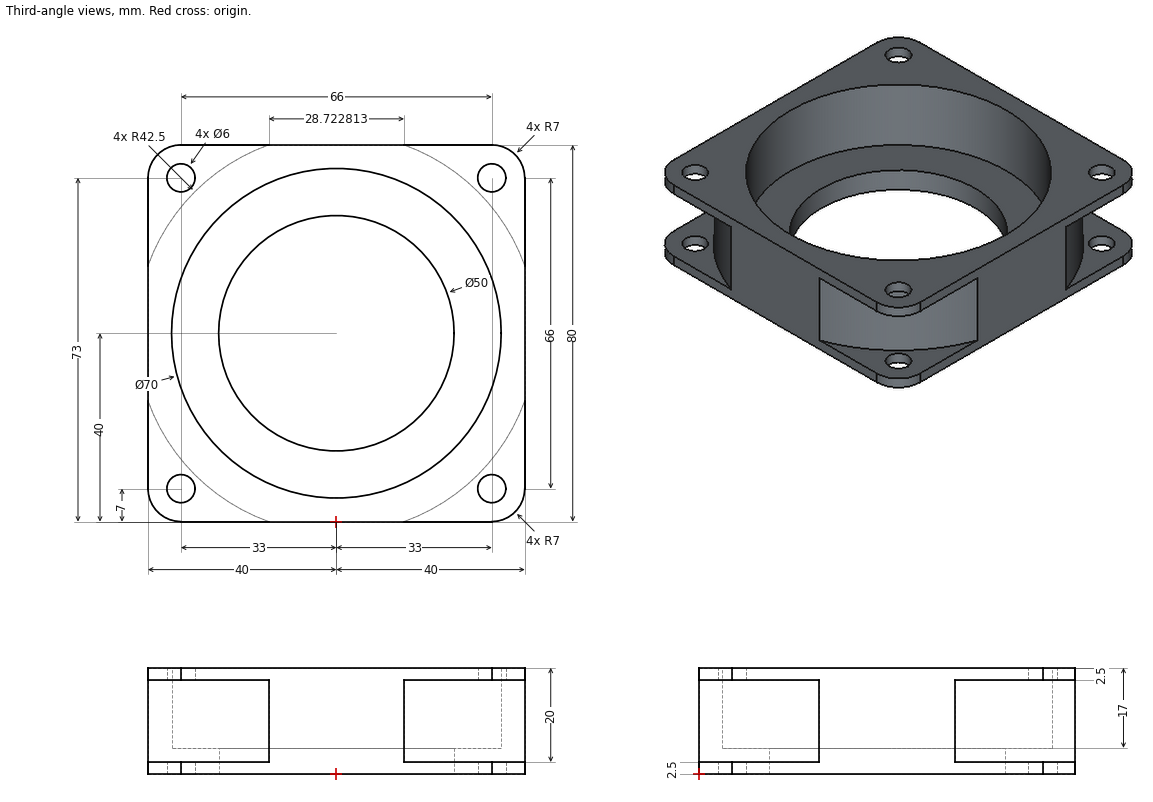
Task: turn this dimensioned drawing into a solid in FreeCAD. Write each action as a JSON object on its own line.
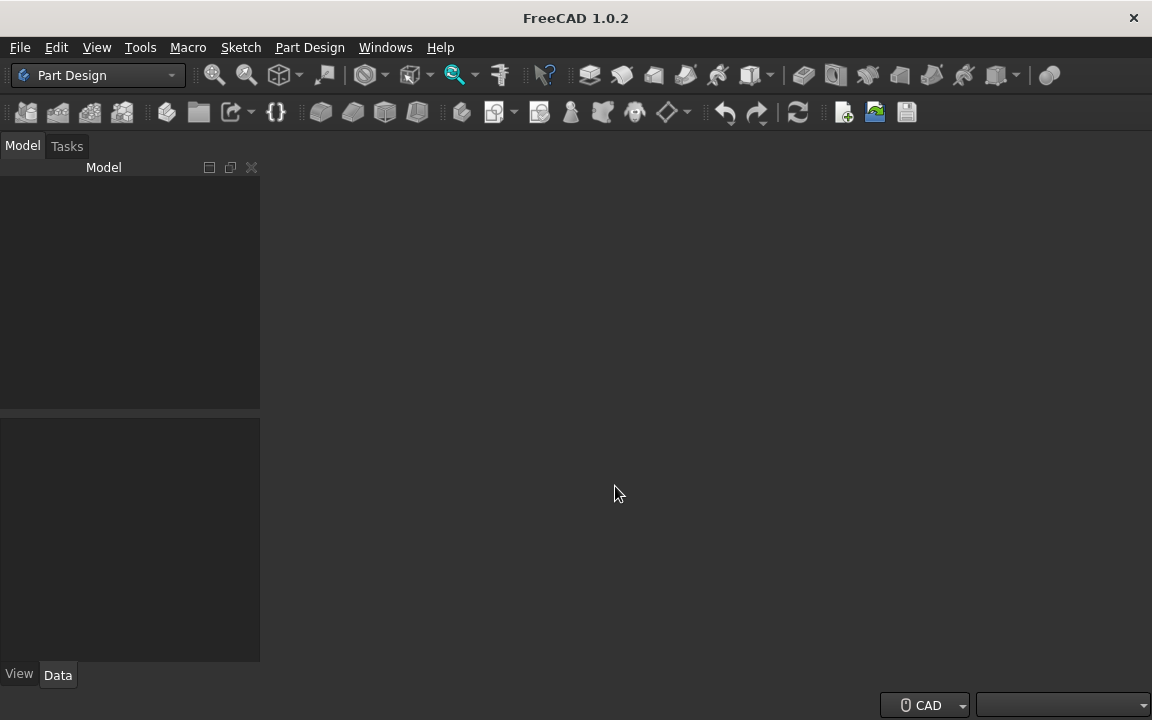
{"action": "left_click", "coordinate": [844, 112]}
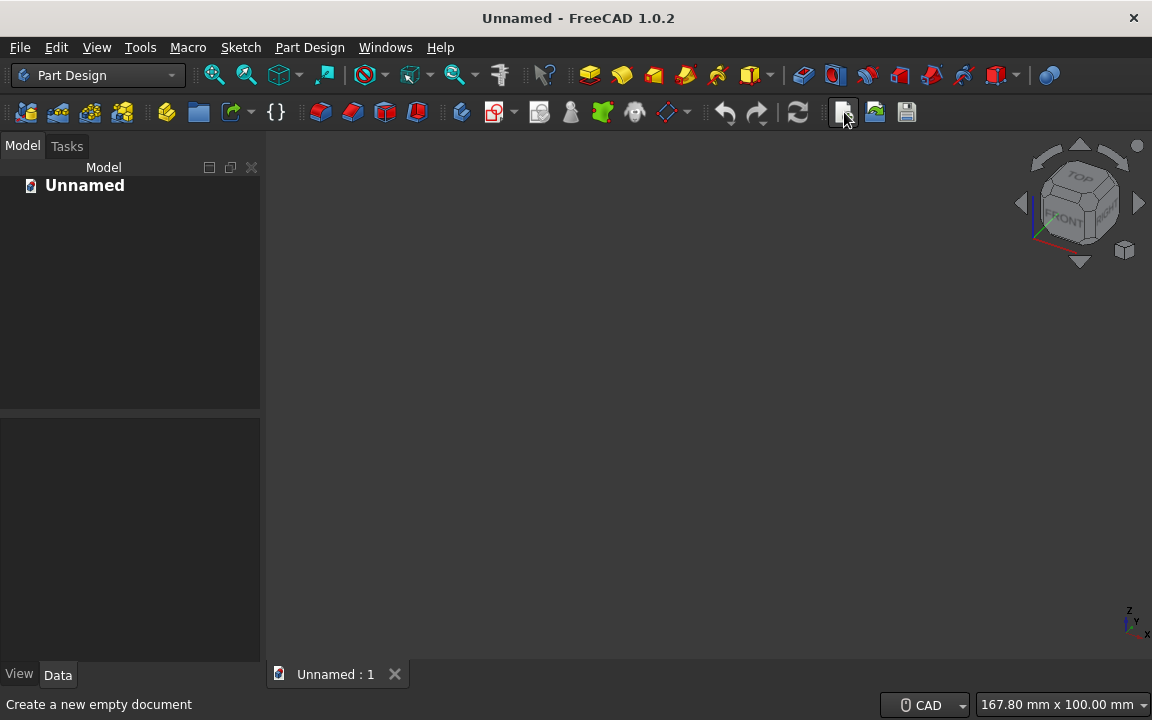
{"action": "left_click", "coordinate": [494, 112]}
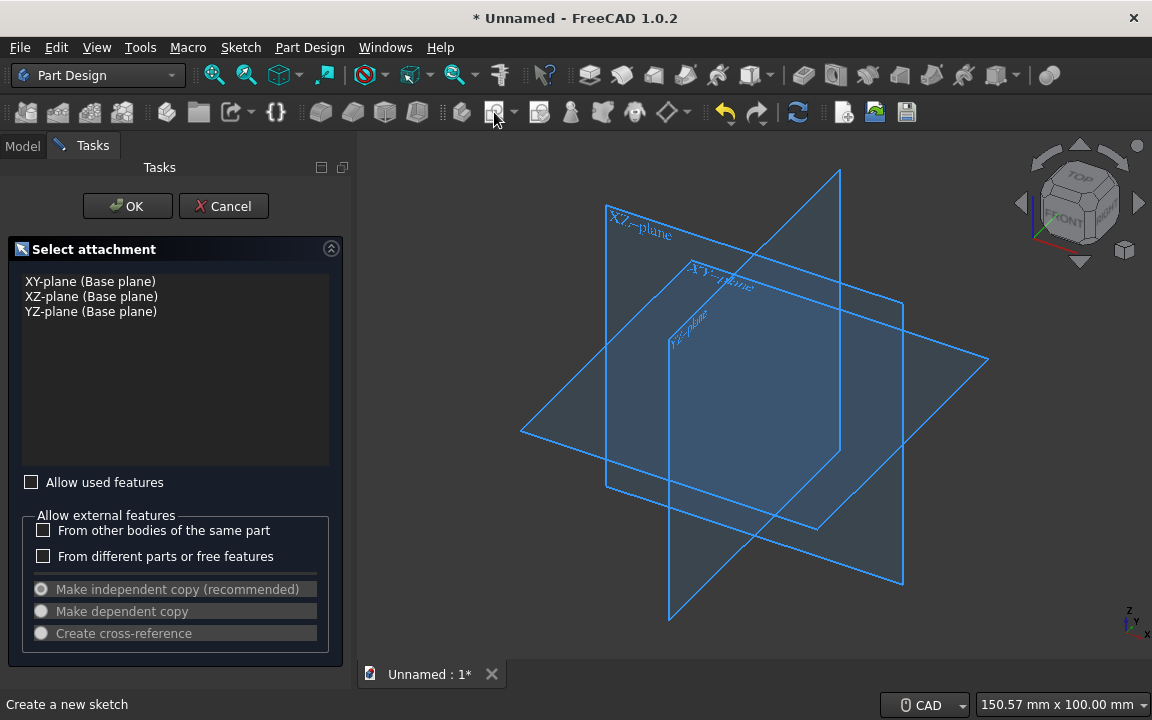
{"action": "left_click", "coordinate": [82, 282]}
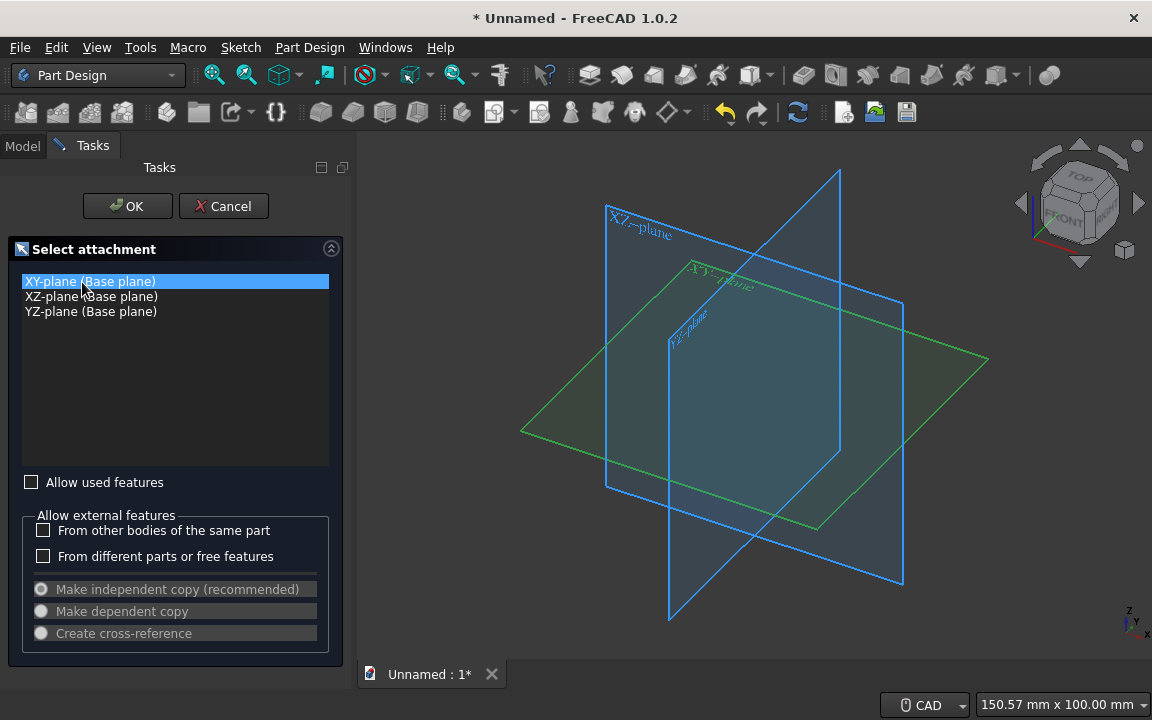
{"action": "left_click", "coordinate": [128, 206]}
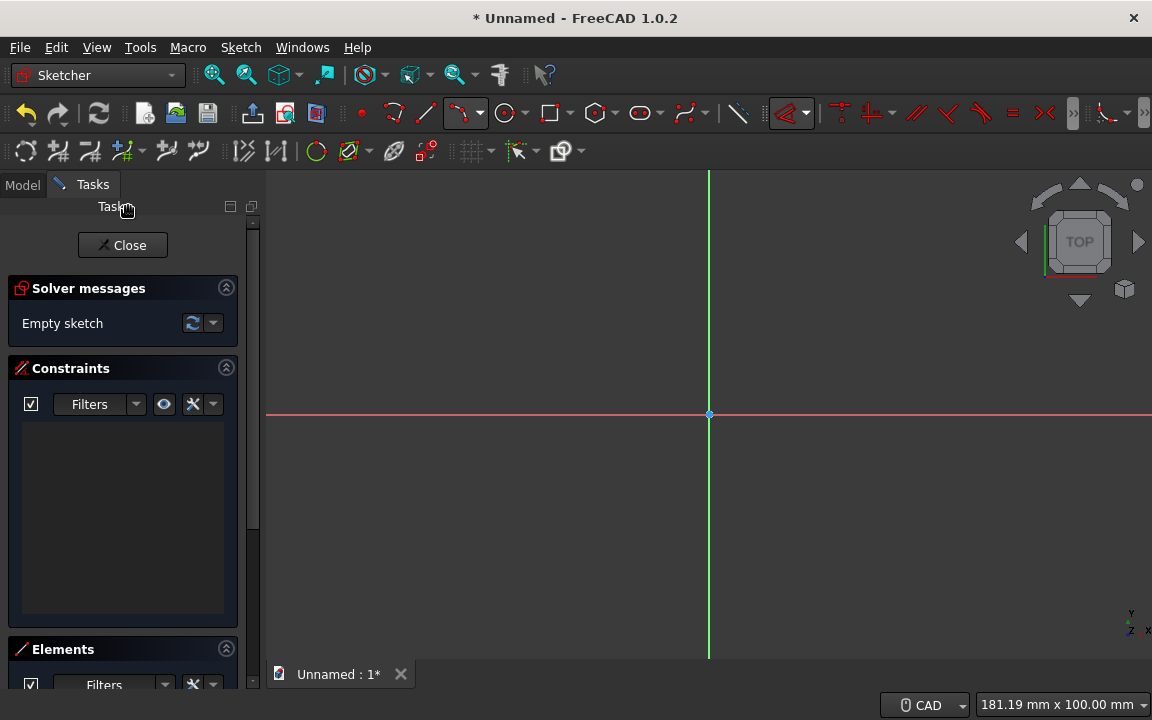
{"action": "scroll", "coordinate": [501, 631], "scroll_direction": "down", "scroll_amount": 2}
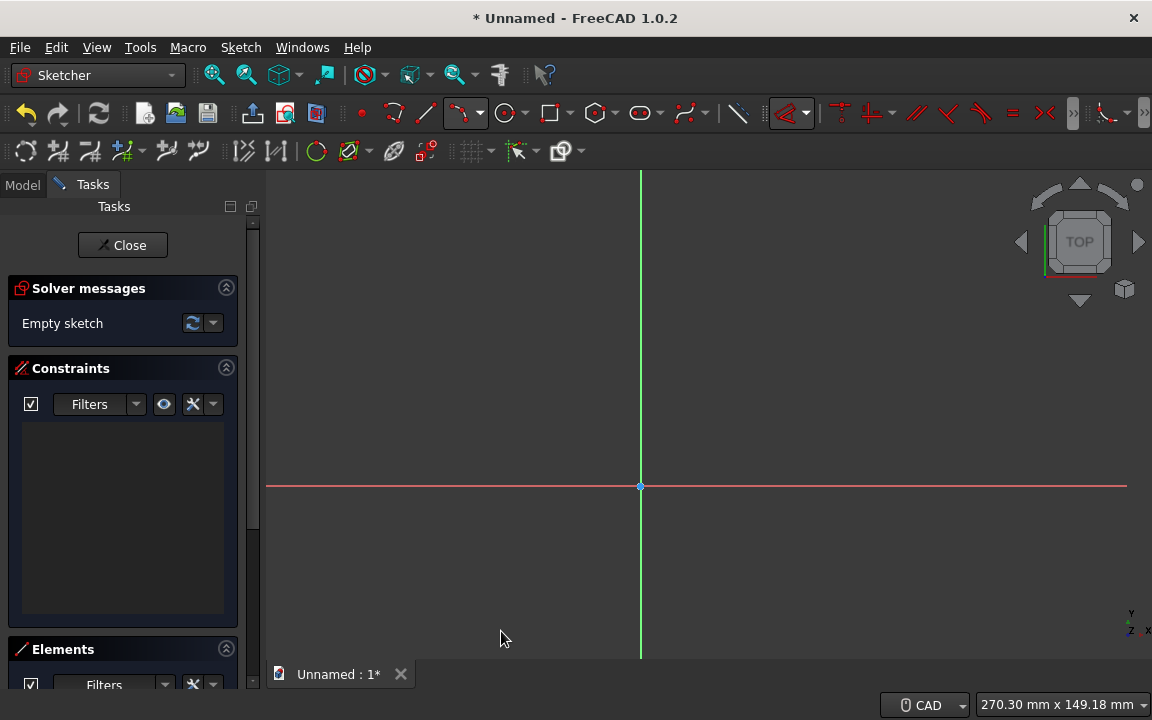
{"action": "left_click", "coordinate": [426, 114]}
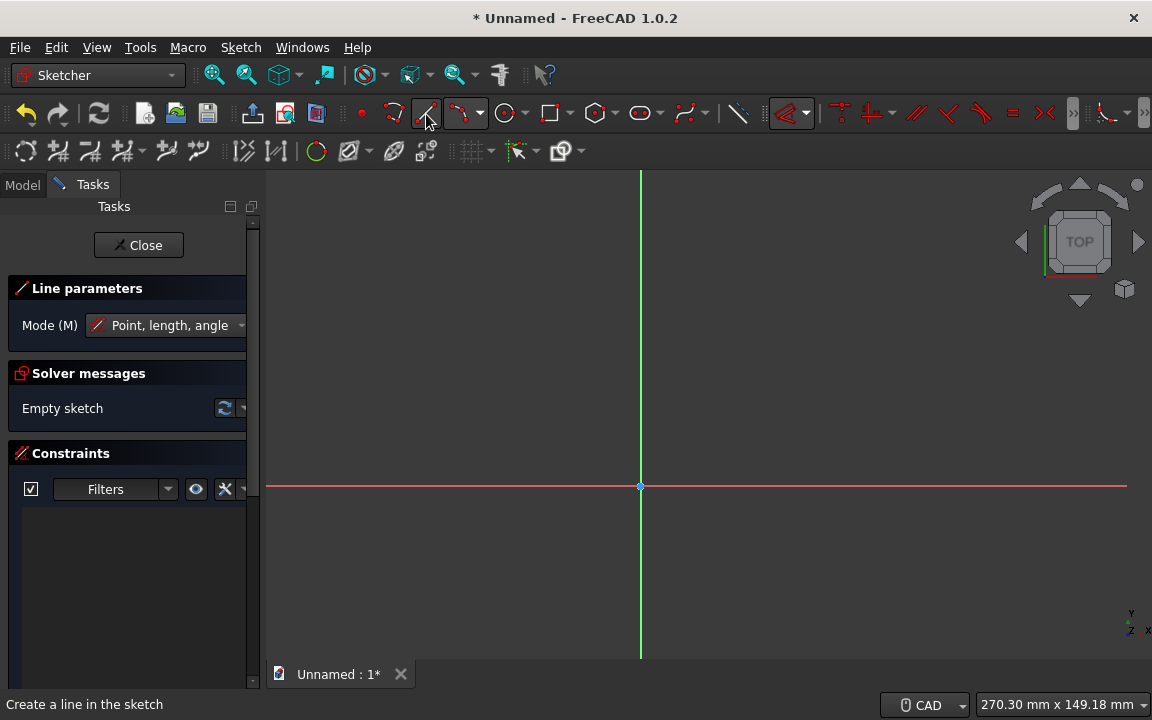
{"action": "left_click", "coordinate": [772, 463]}
{"action": "left_click", "coordinate": [772, 247]}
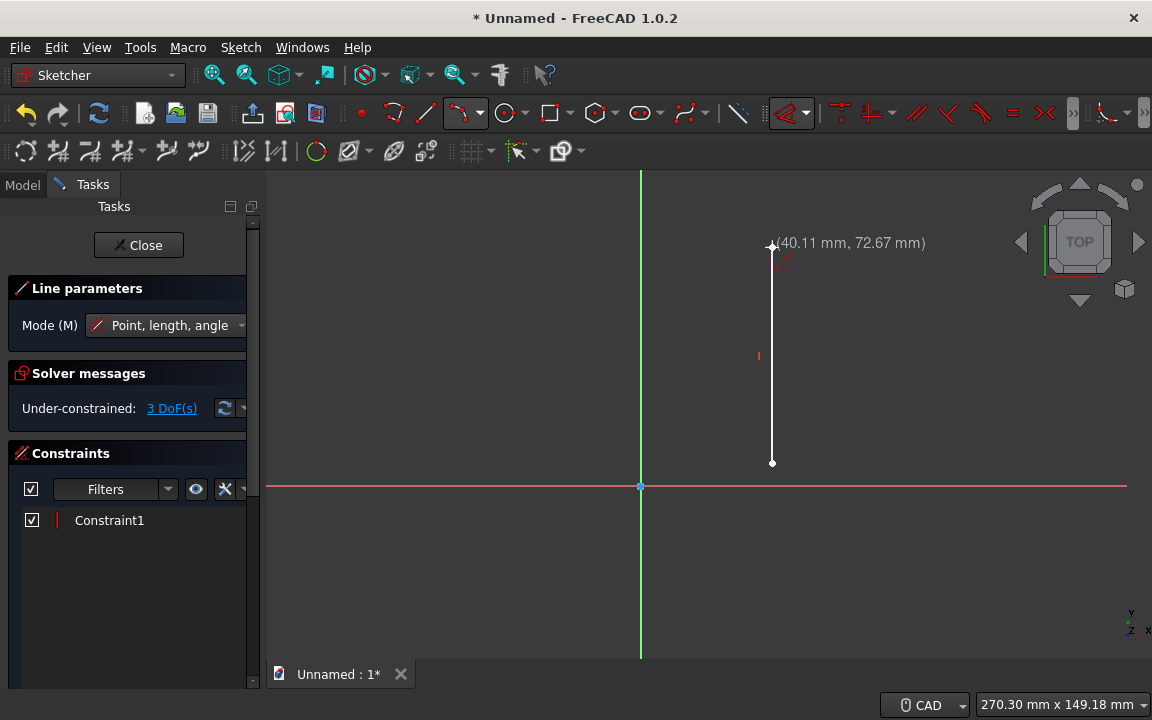
{"action": "left_click", "coordinate": [749, 224]}
{"action": "left_click", "coordinate": [532, 224]}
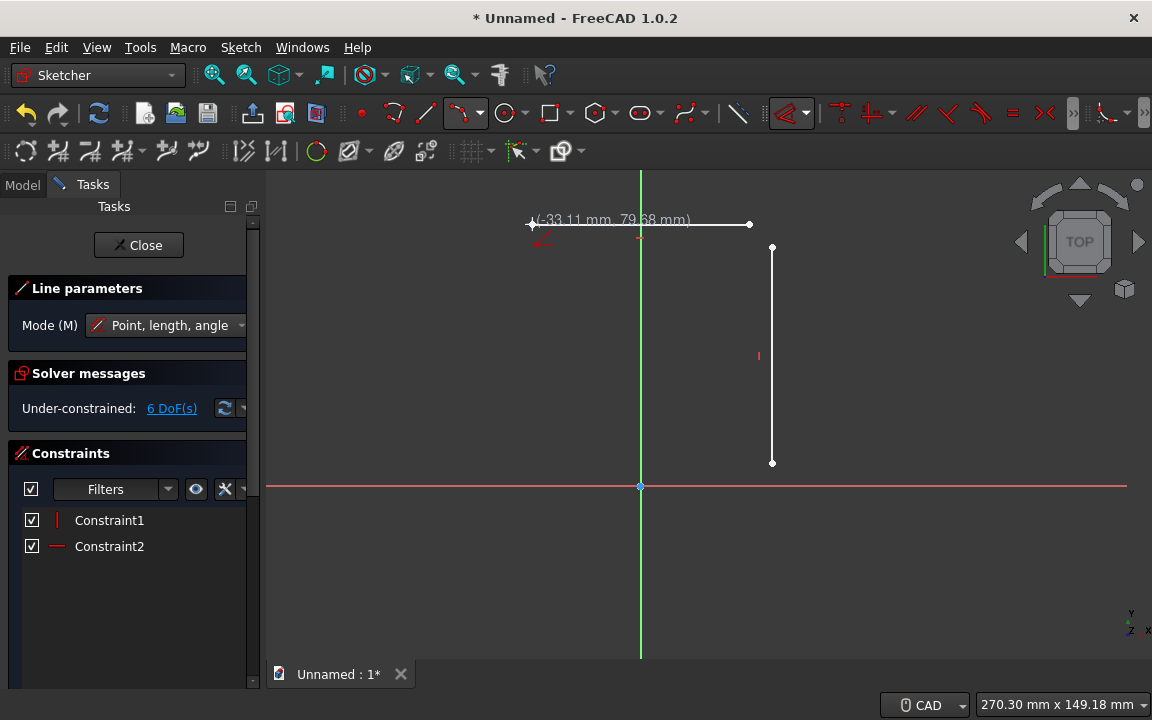
{"action": "left_click", "coordinate": [509, 247]}
{"action": "left_click", "coordinate": [509, 463]}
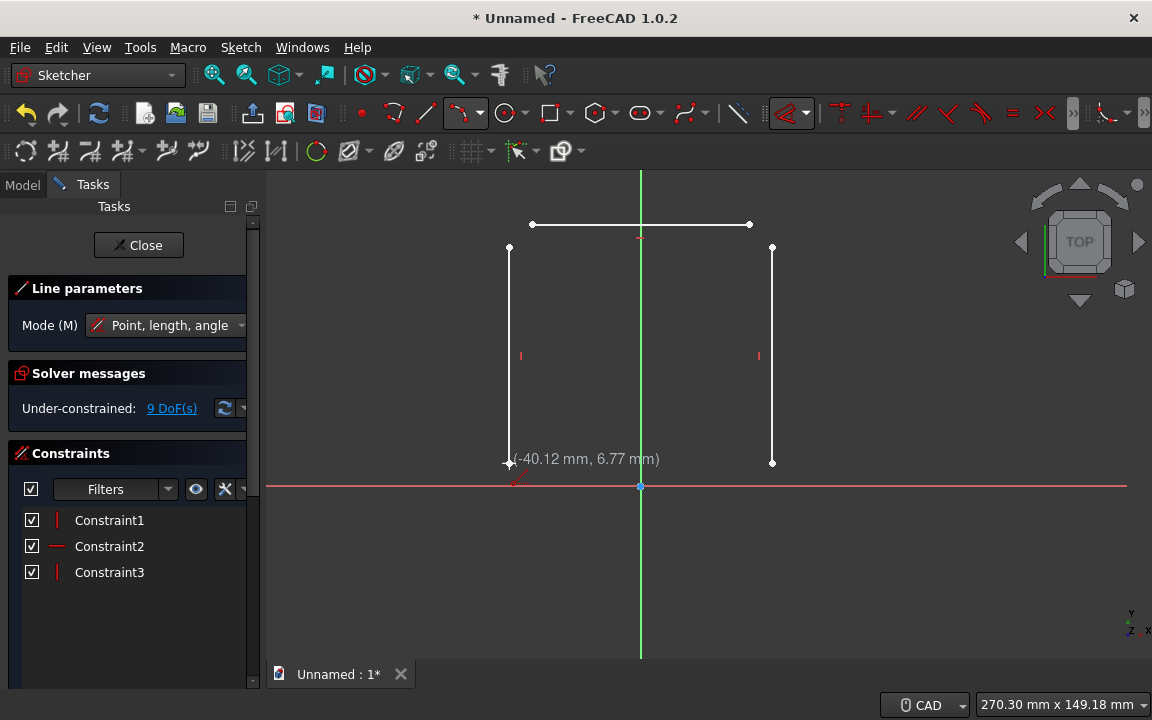
{"action": "left_click", "coordinate": [532, 486]}
{"action": "left_click", "coordinate": [749, 477]}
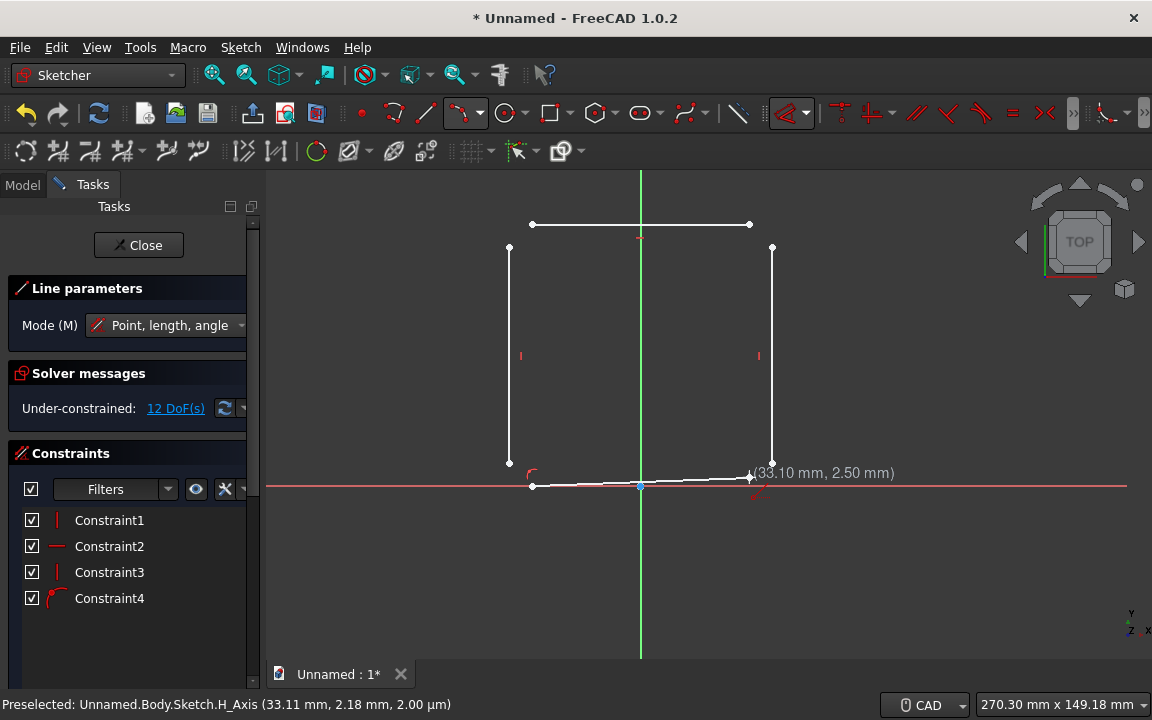
{"action": "left_click", "coordinate": [460, 114]}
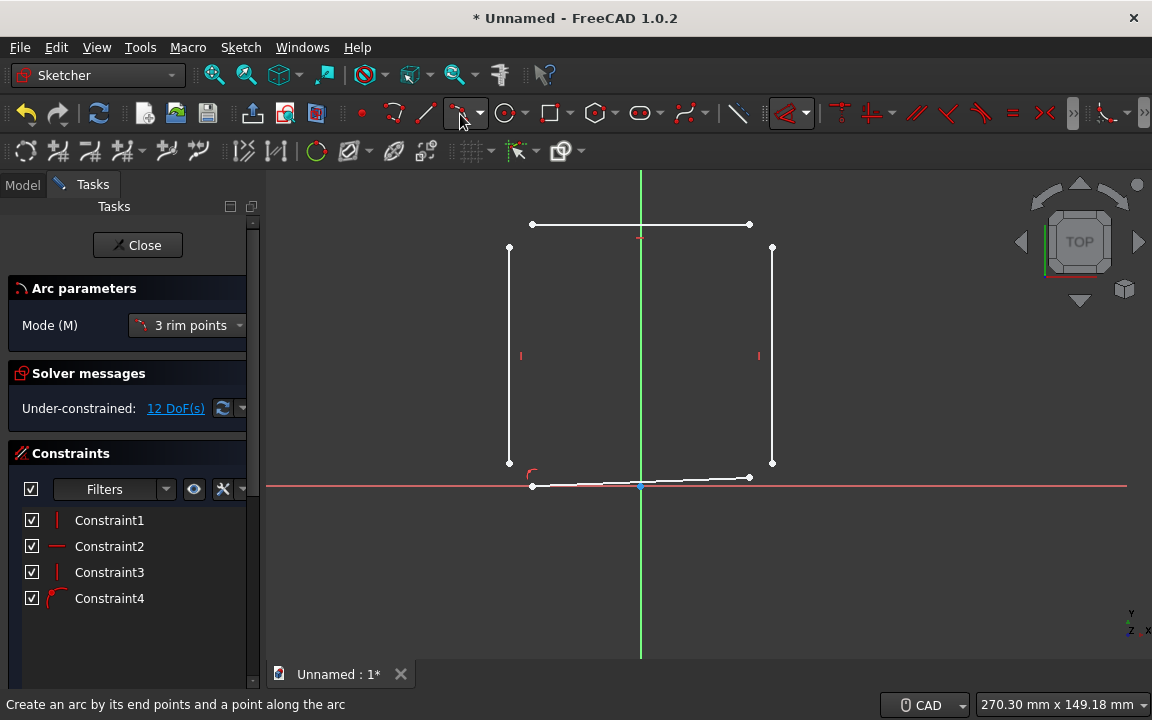
{"action": "left_click", "coordinate": [772, 248]}
{"action": "left_click", "coordinate": [749, 225]}